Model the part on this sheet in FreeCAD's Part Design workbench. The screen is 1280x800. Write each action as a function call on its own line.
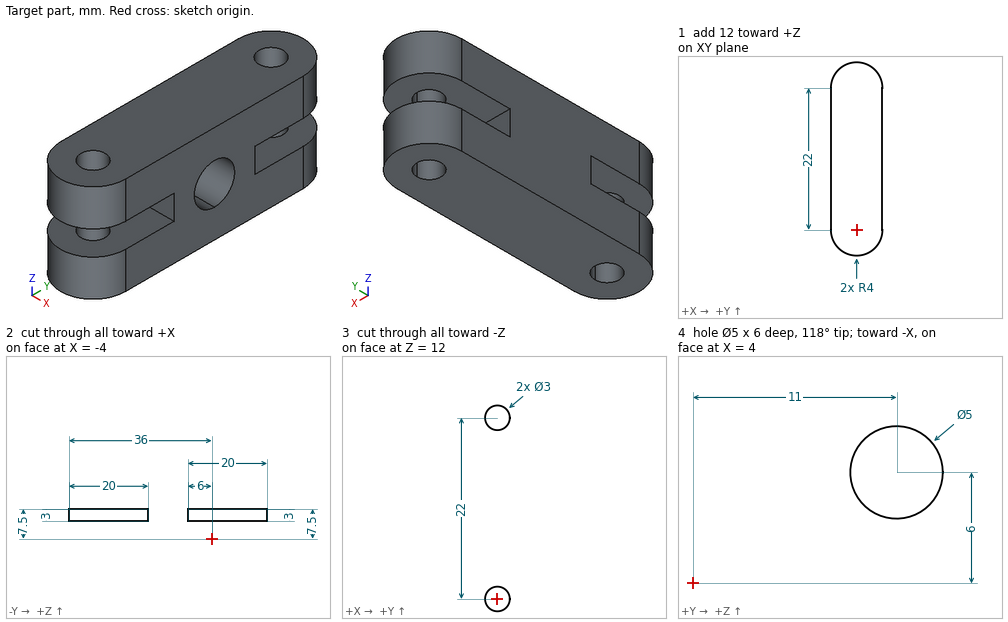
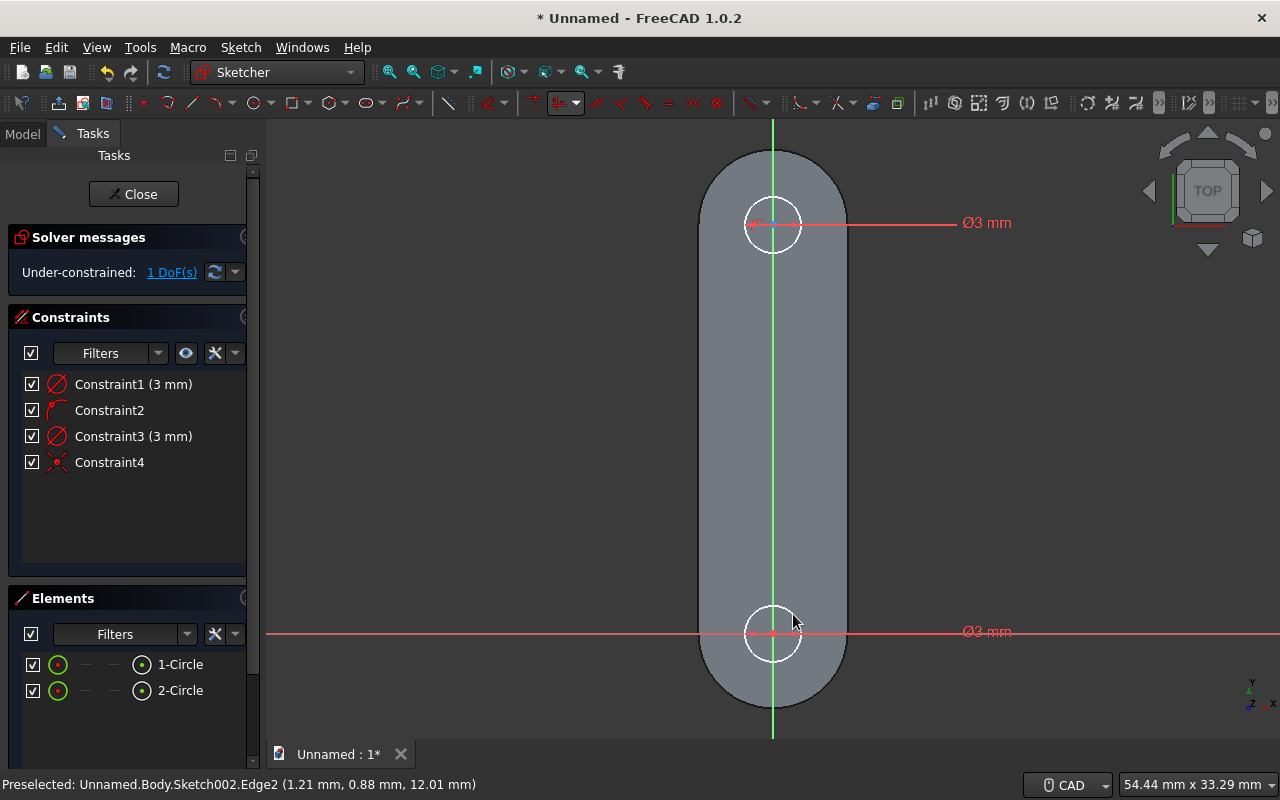
key(d)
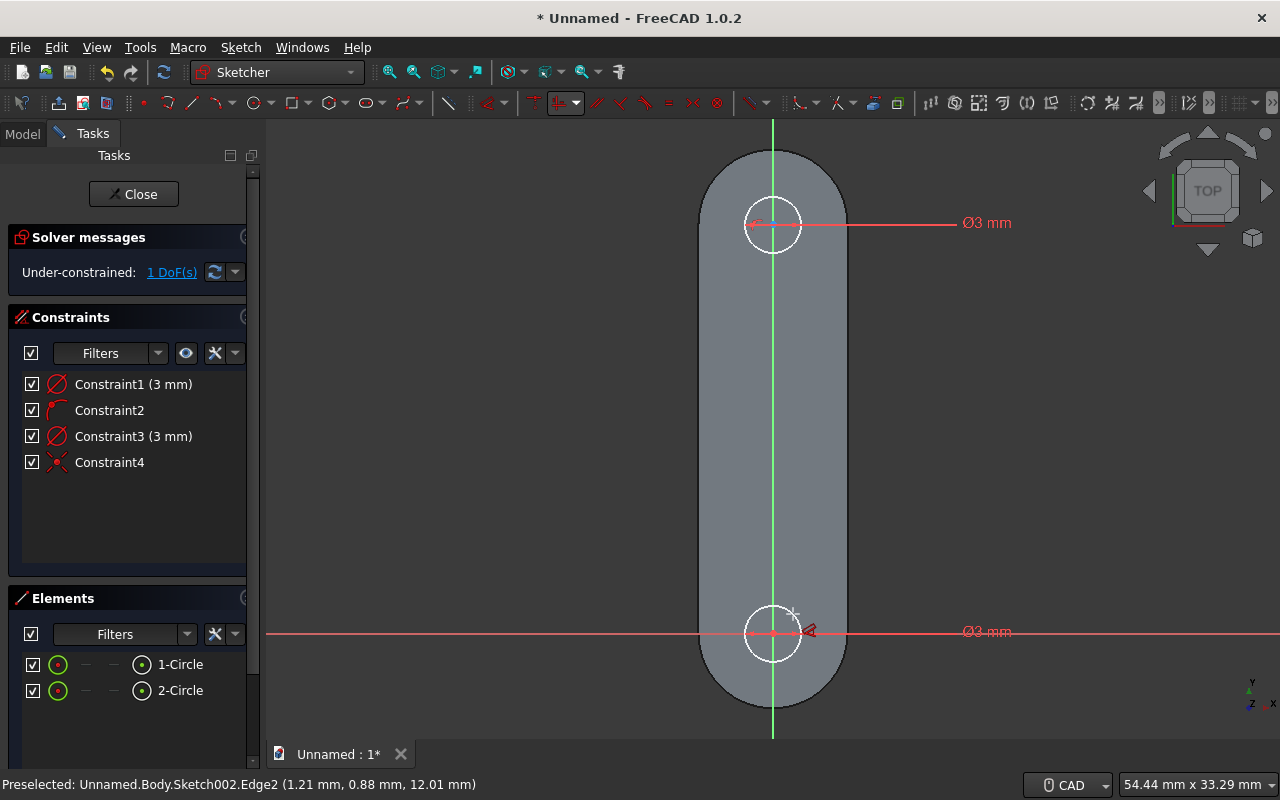
click(773, 225)
click(807, 429)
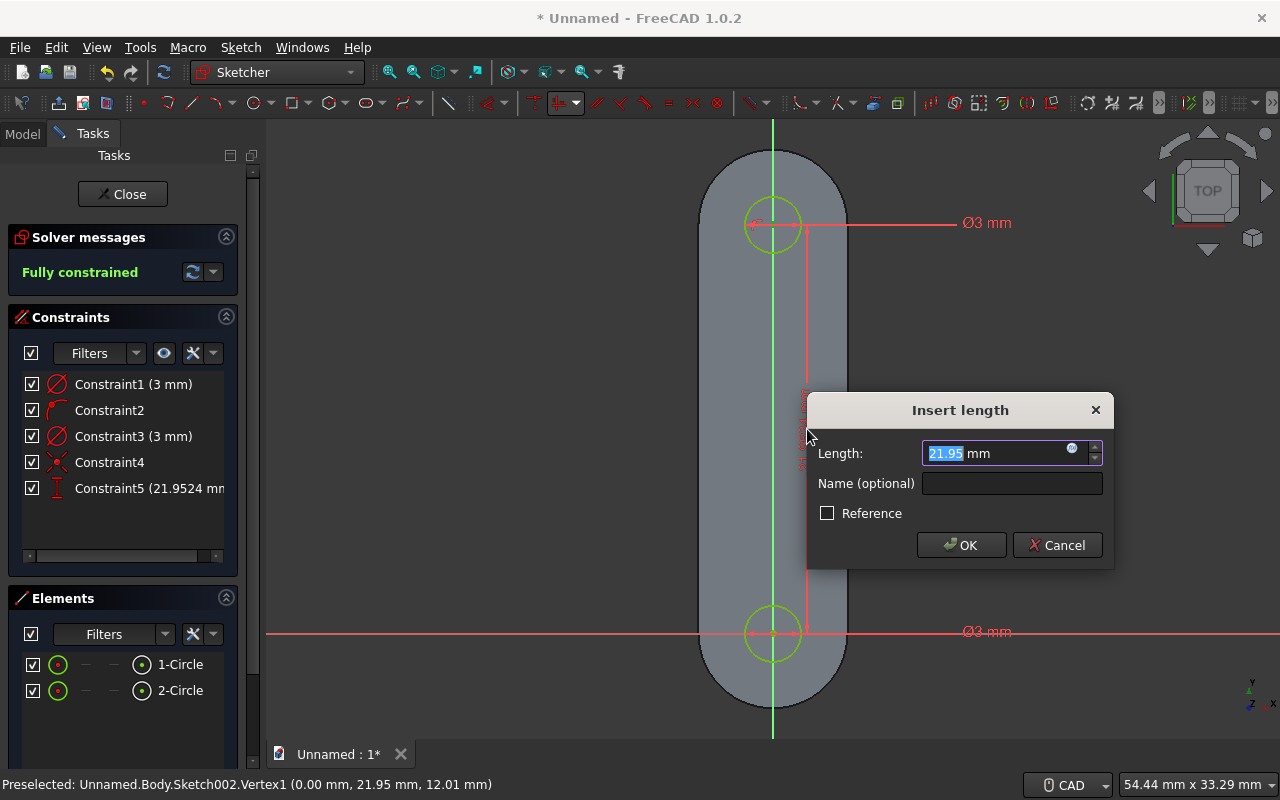
text(22)
key(Return)
key(Escape)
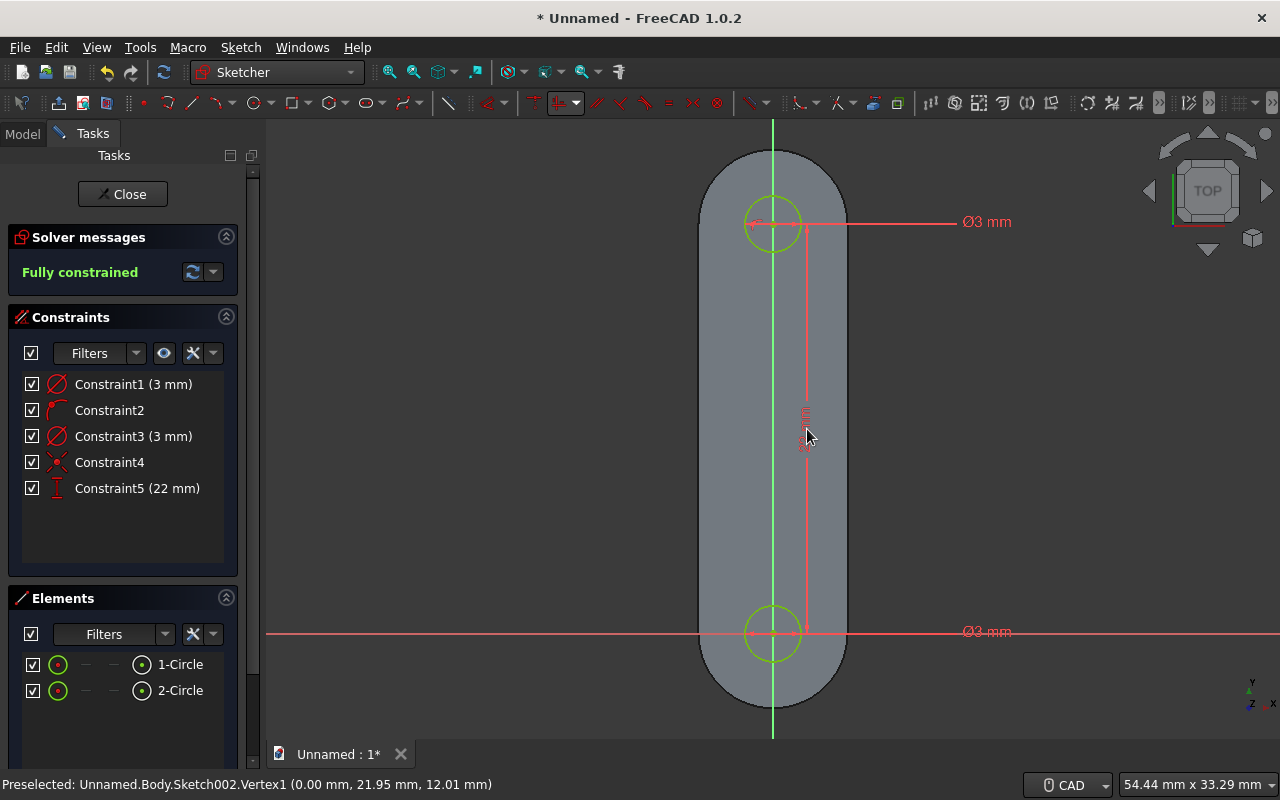
click(123, 194)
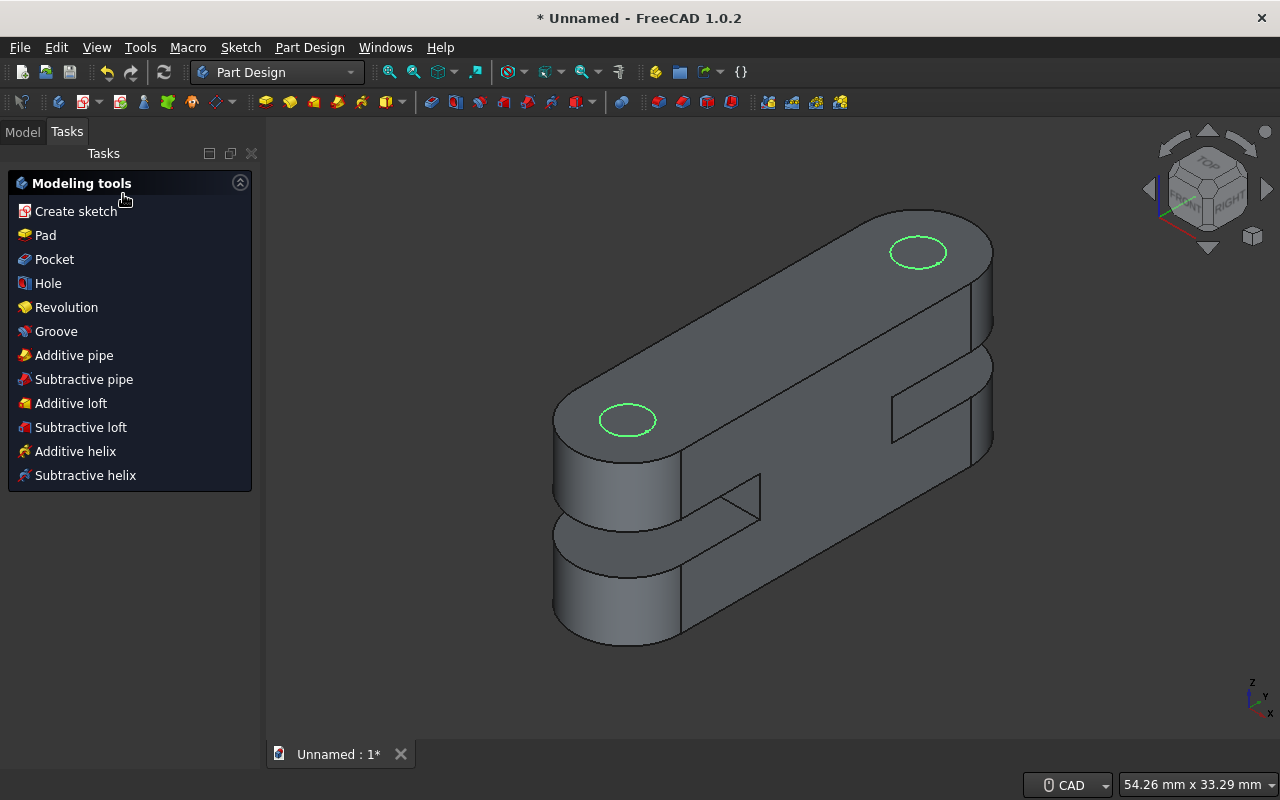
click(432, 102)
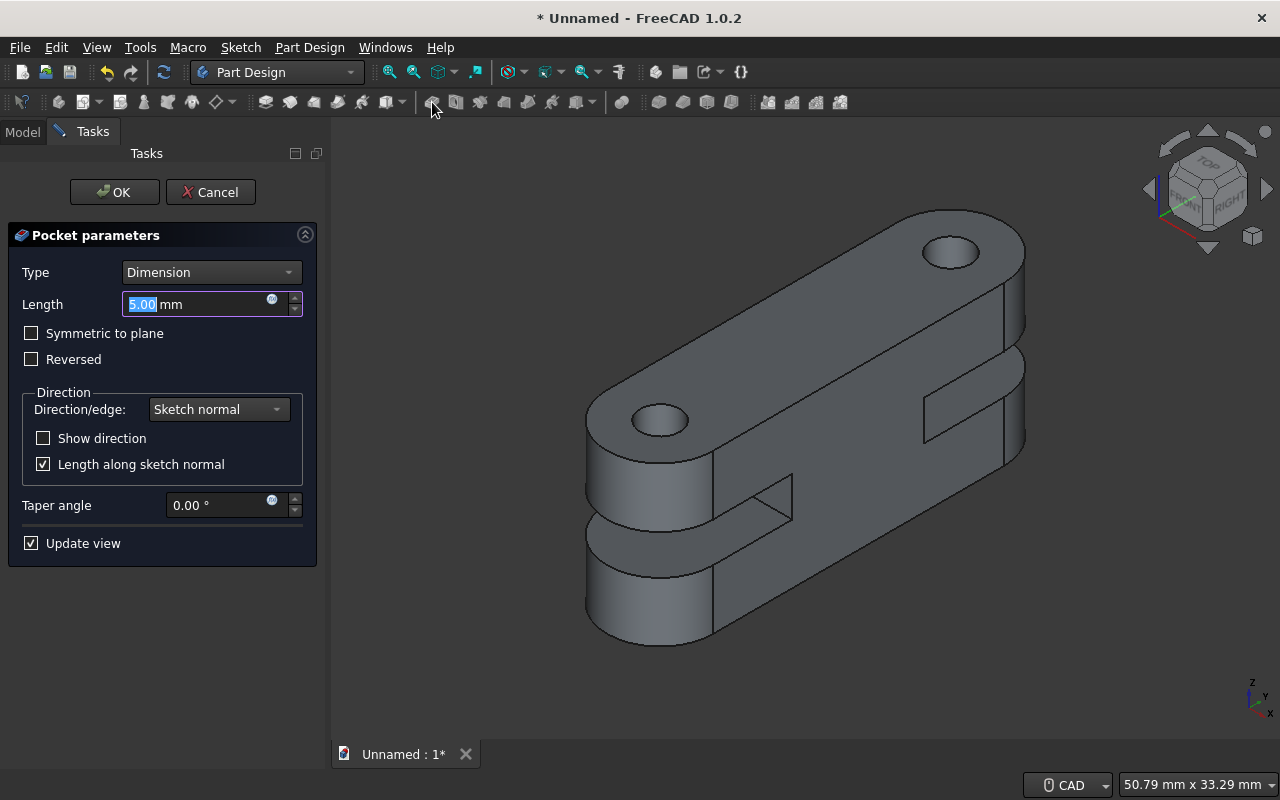
click(212, 272)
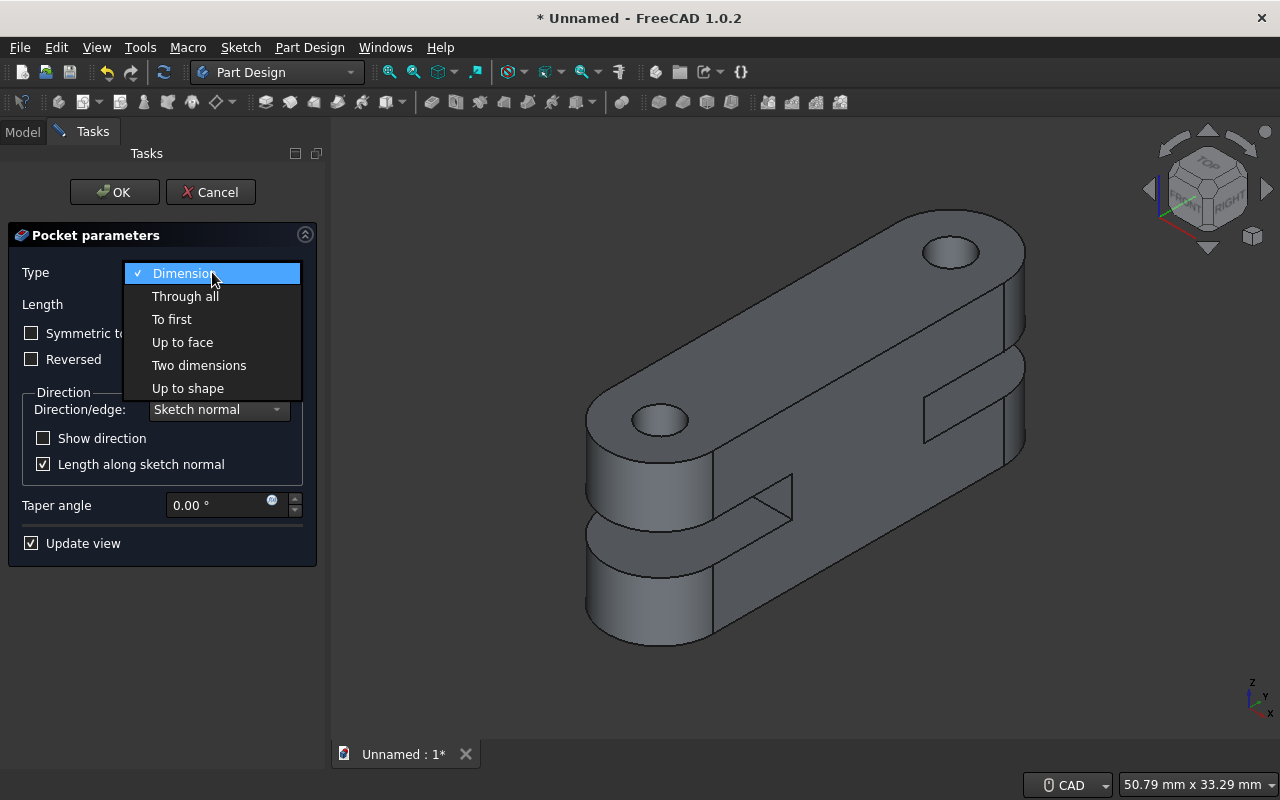
click(212, 296)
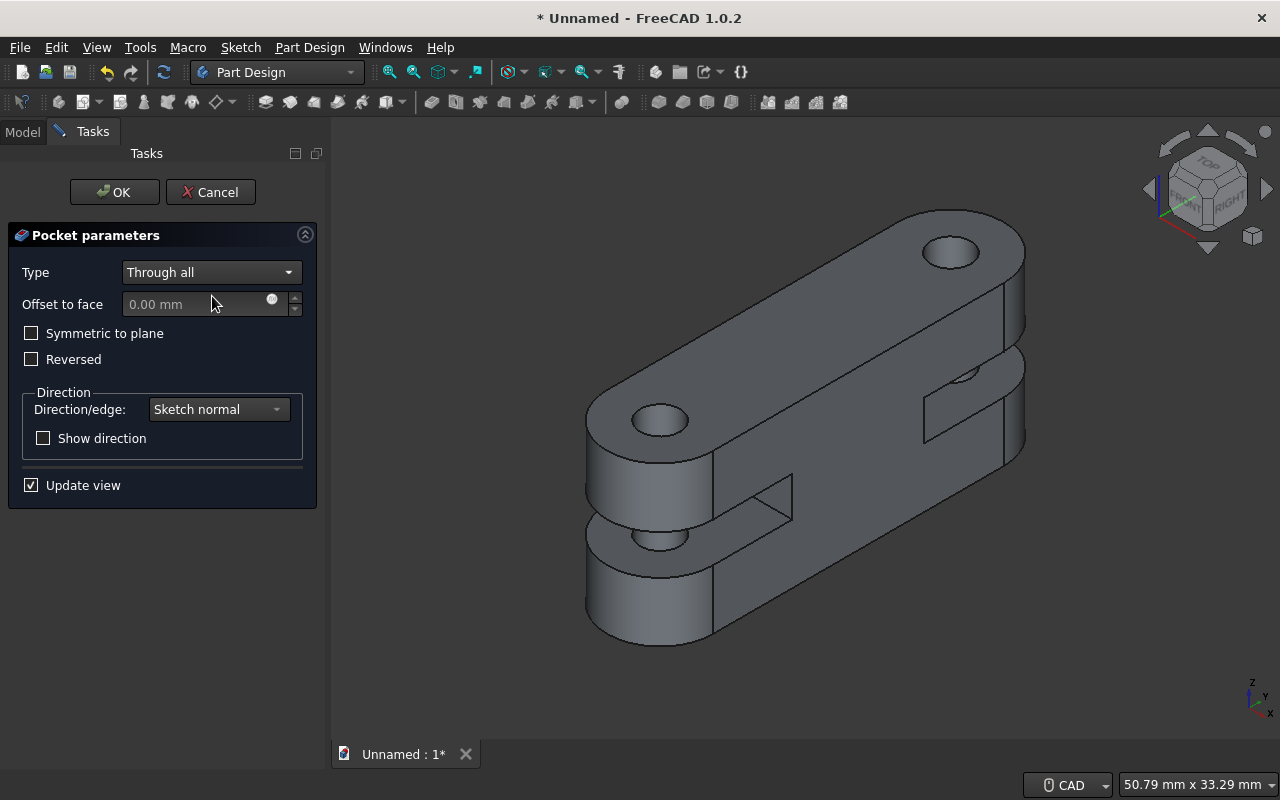
click(115, 192)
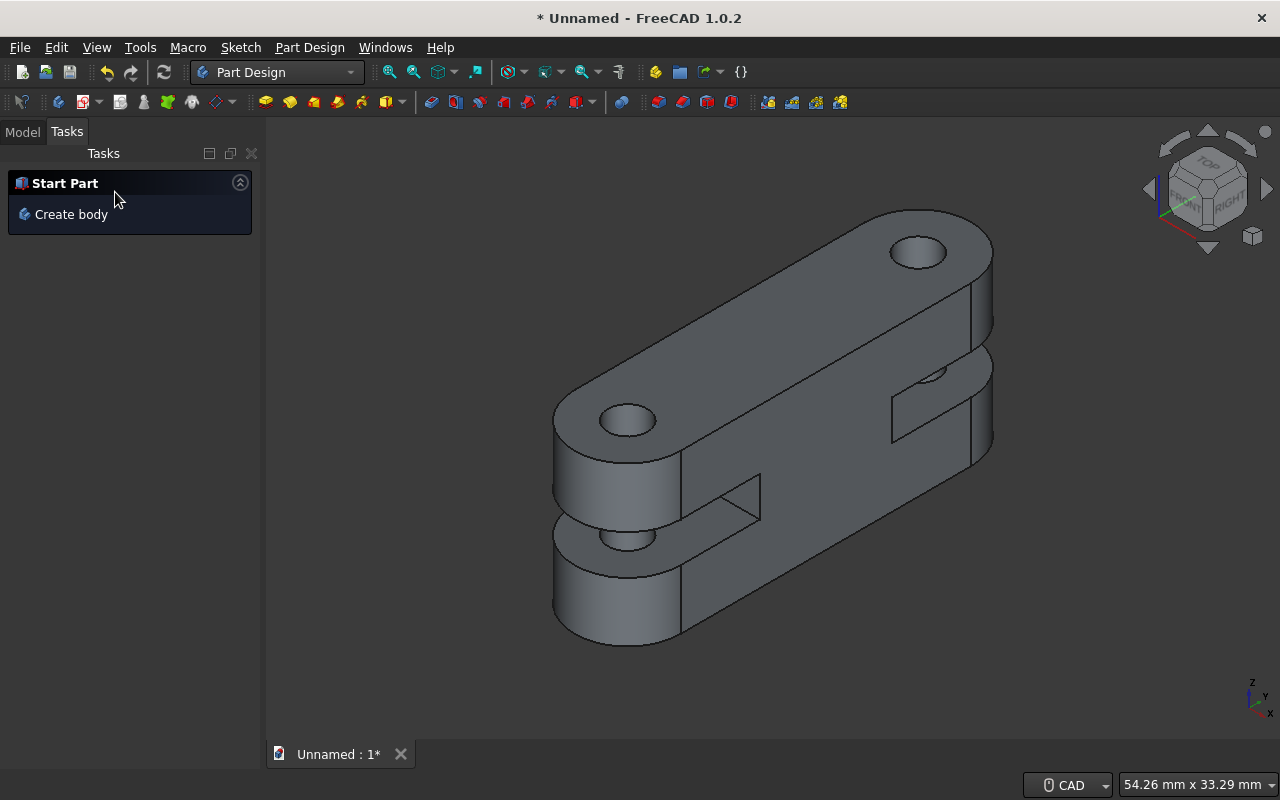
click(826, 458)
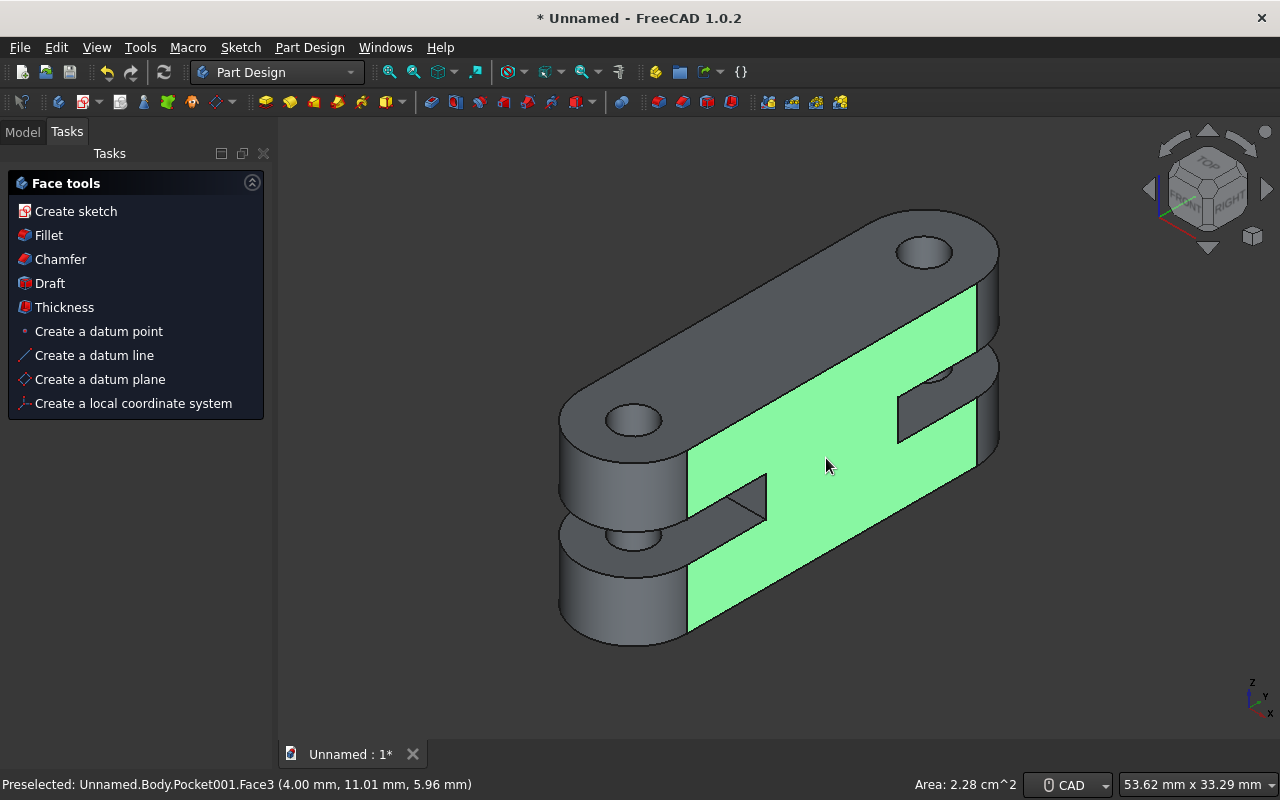
click(84, 102)